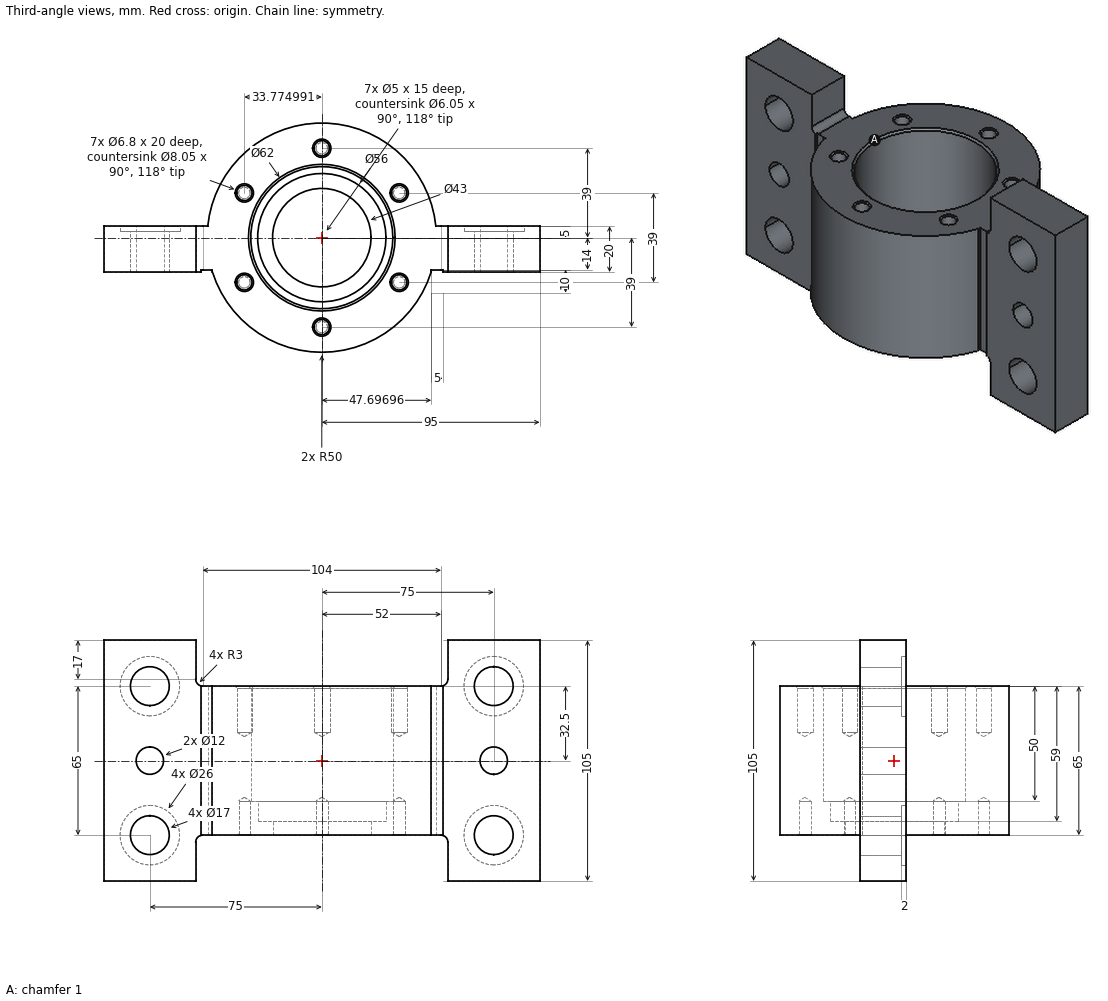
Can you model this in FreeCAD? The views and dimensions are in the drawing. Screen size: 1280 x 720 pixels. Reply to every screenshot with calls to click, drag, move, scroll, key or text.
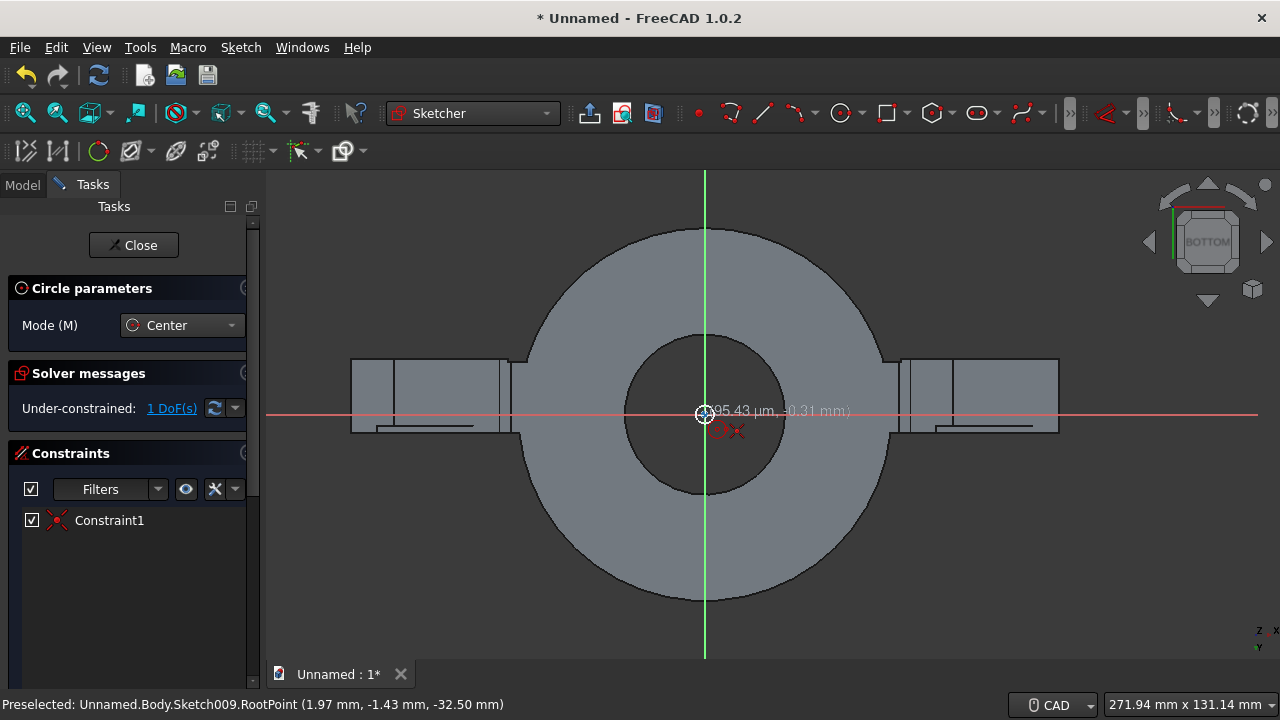
scroll(705, 560, up, 5)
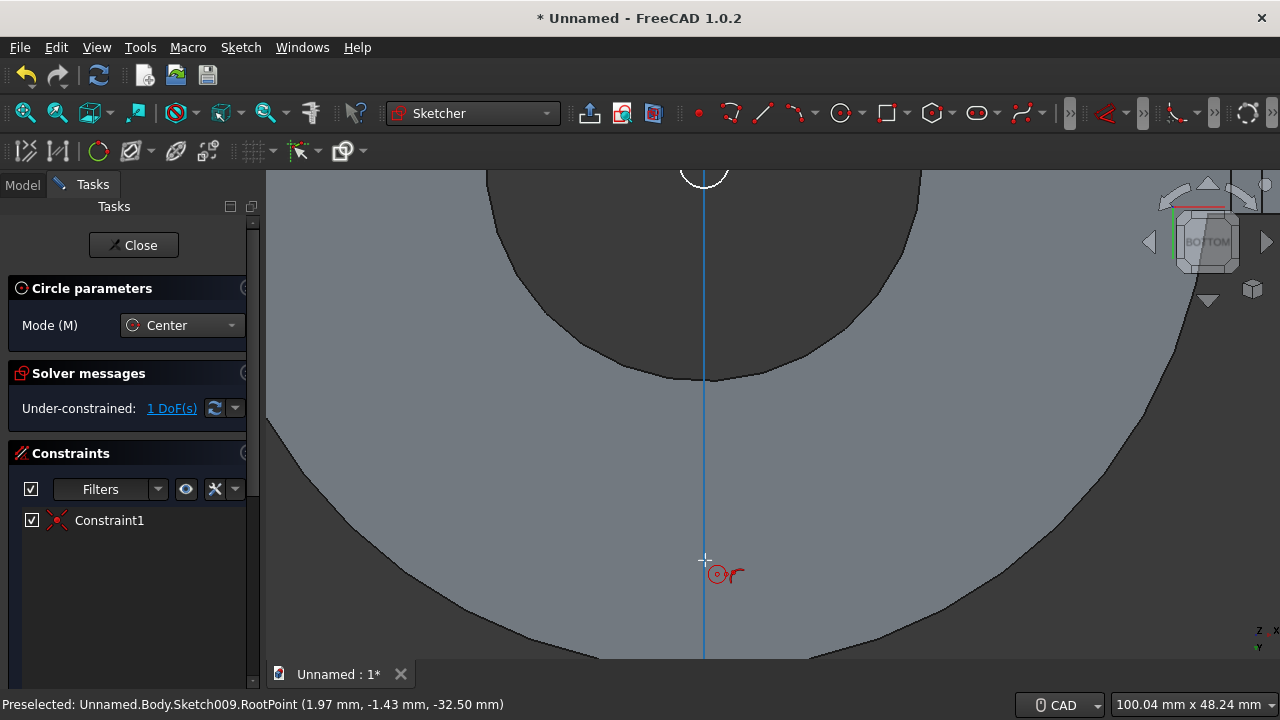
click(704, 559)
click(722, 541)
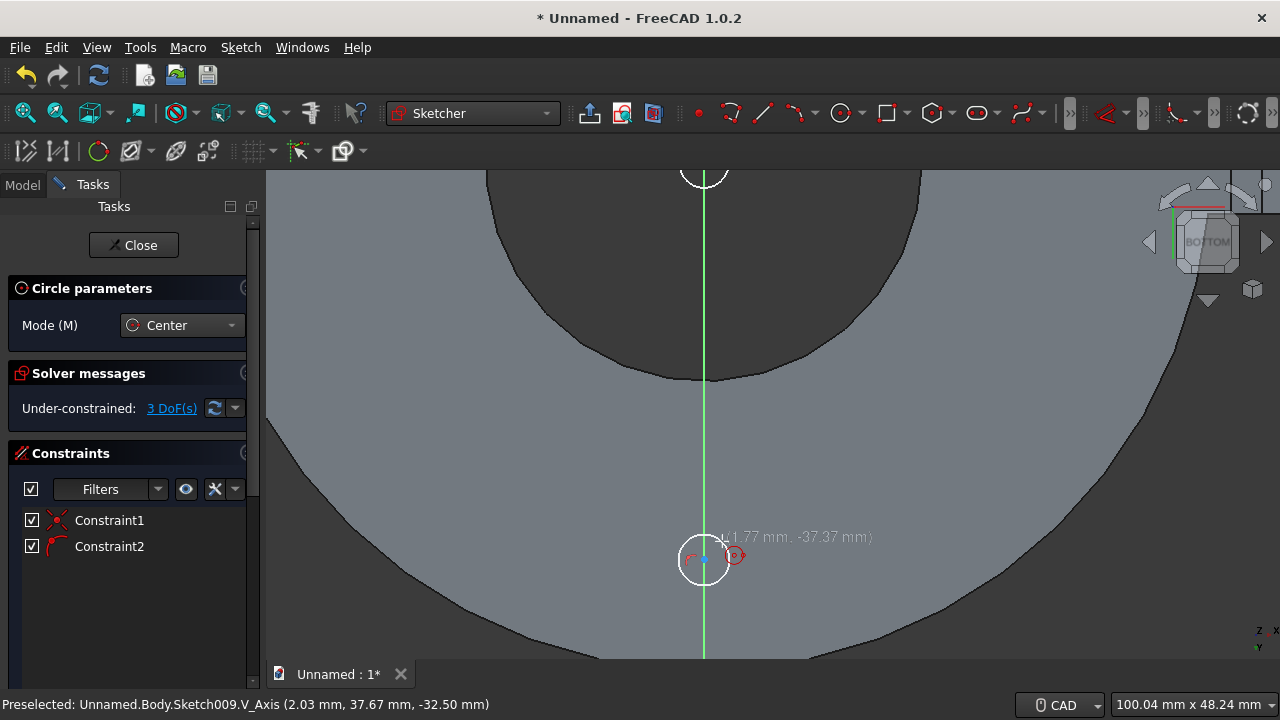
click(362, 361)
click(380, 343)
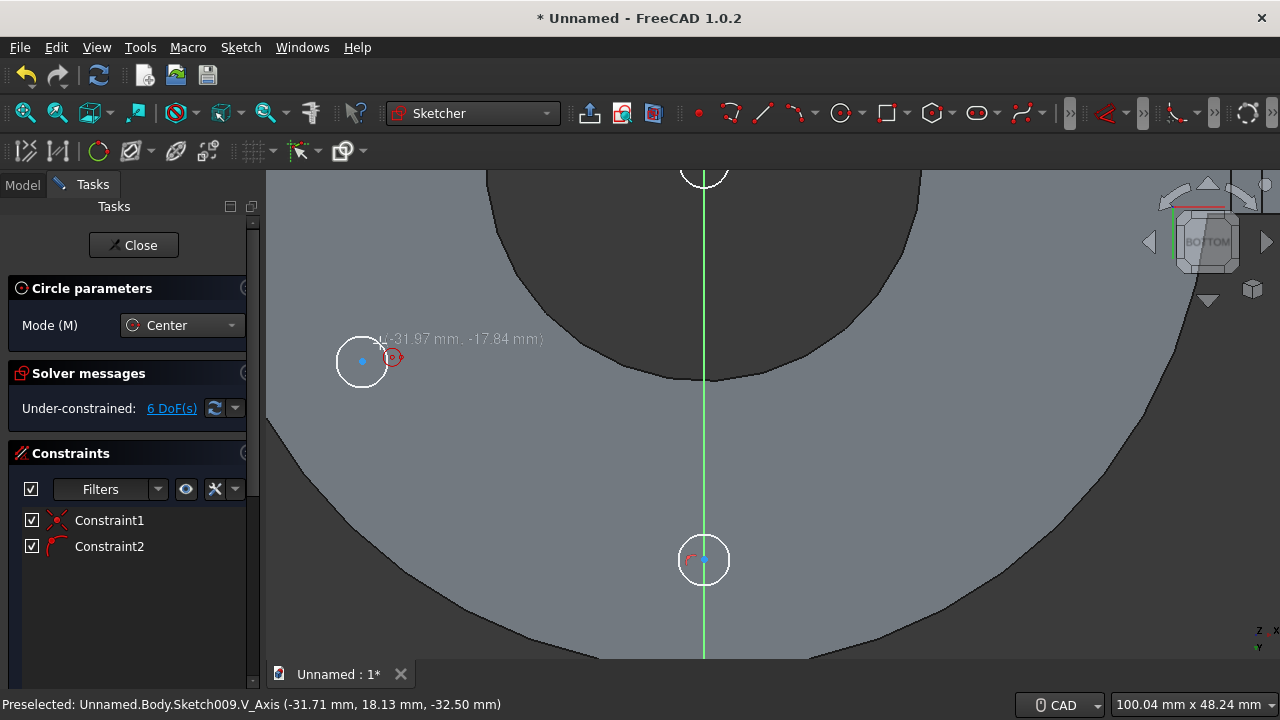
scroll(705, 561, down, 5)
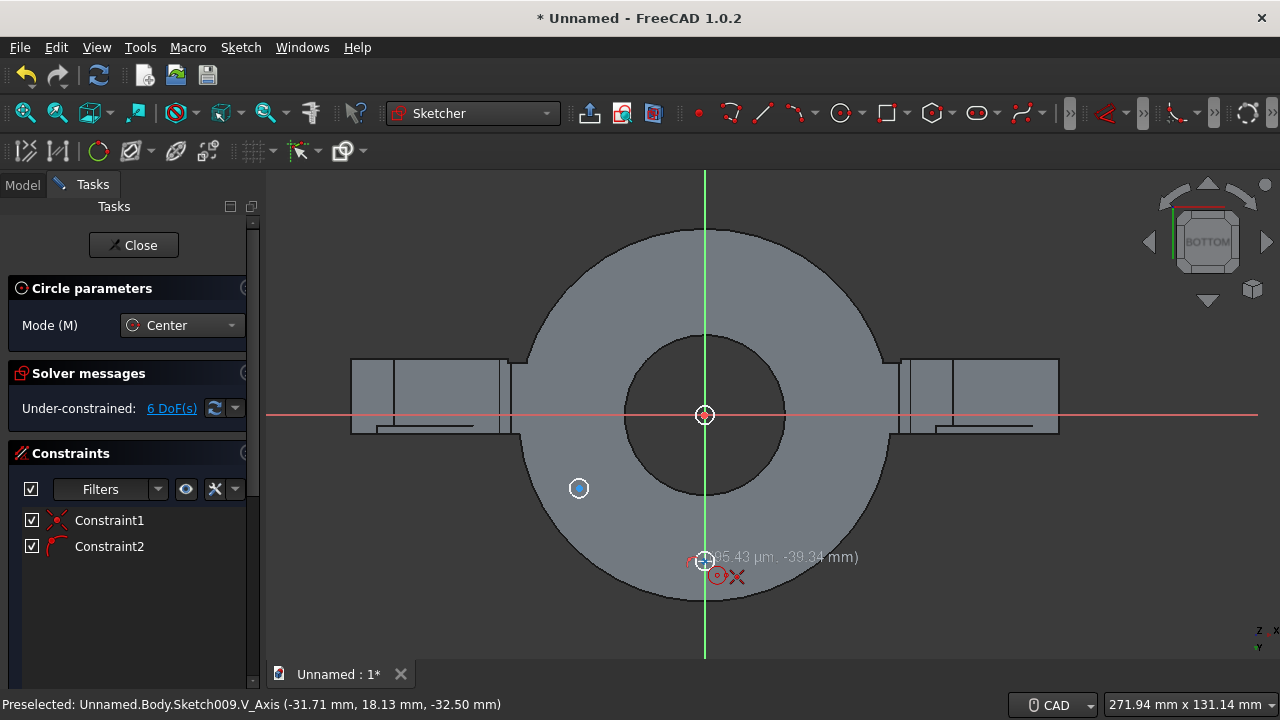
scroll(579, 342, up, 5)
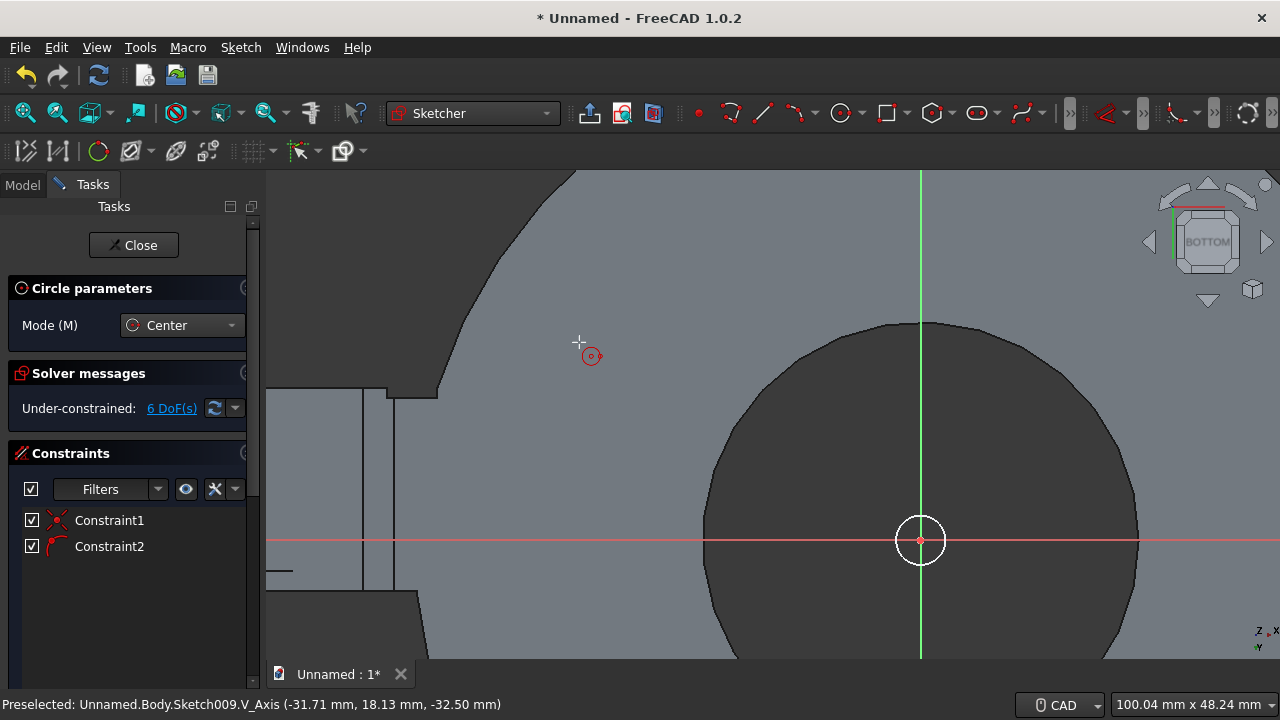
click(578, 343)
click(596, 325)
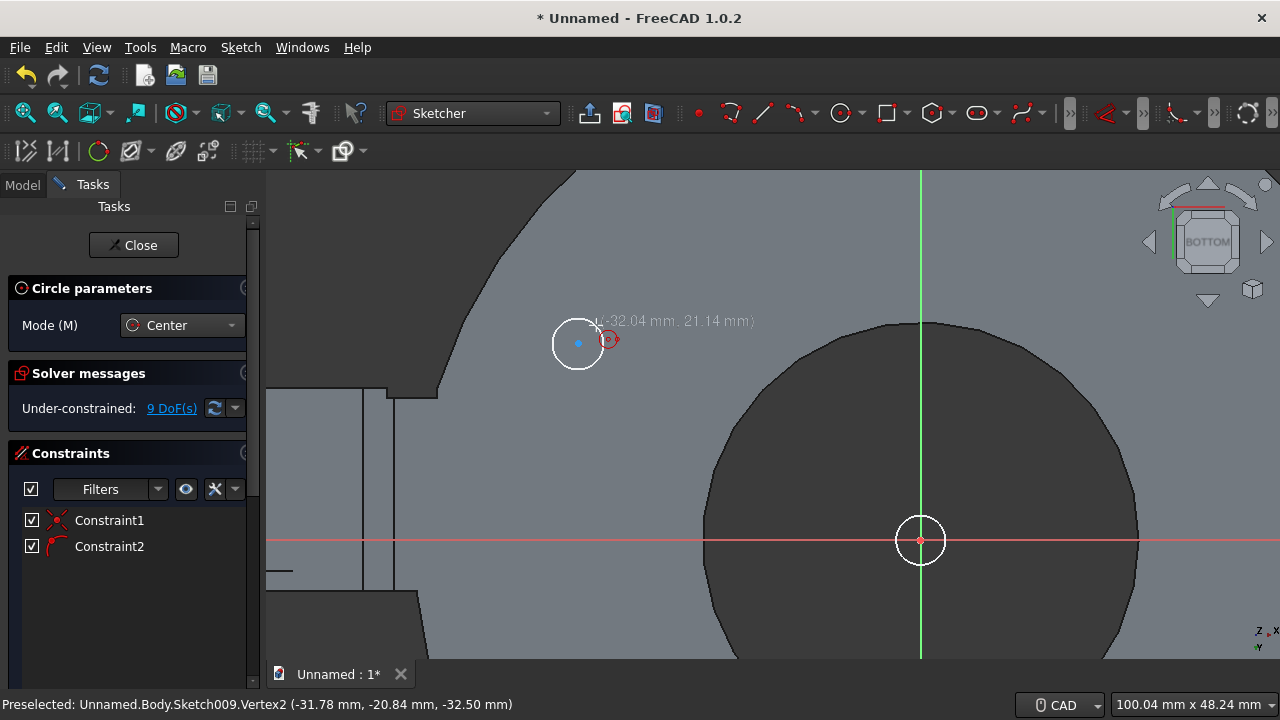
scroll(579, 341, down, 5)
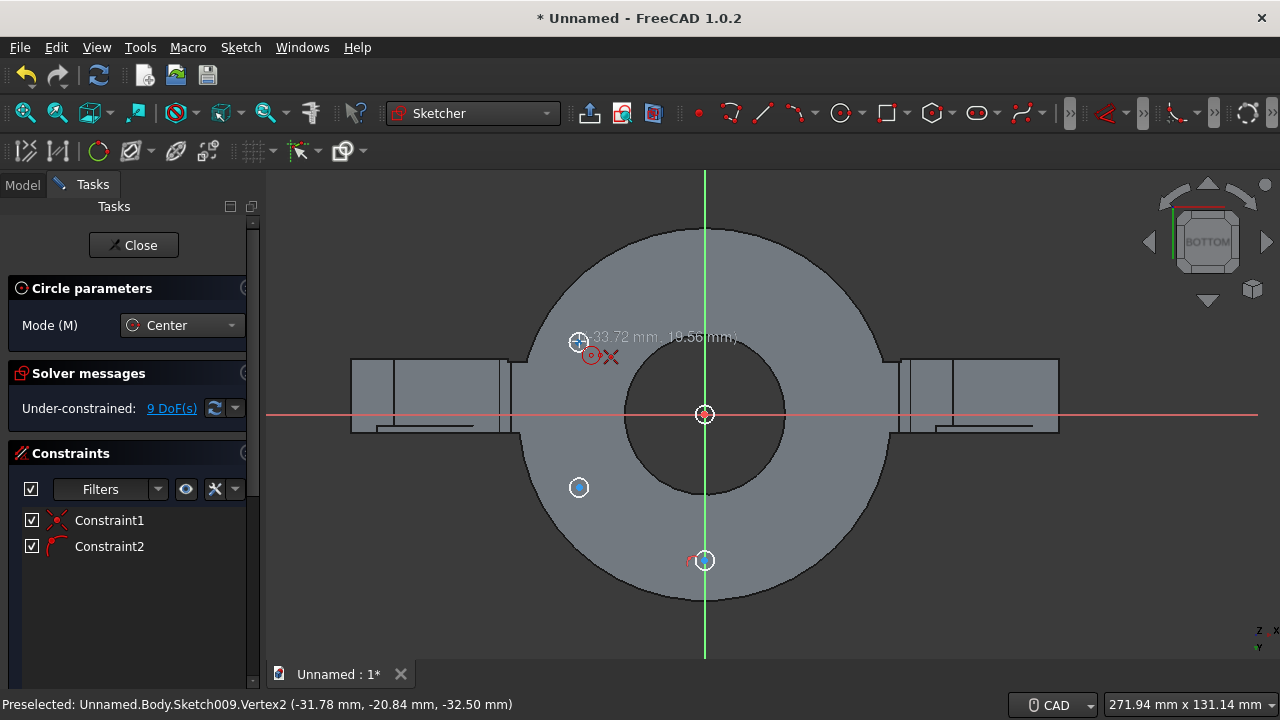
scroll(705, 269, up, 5)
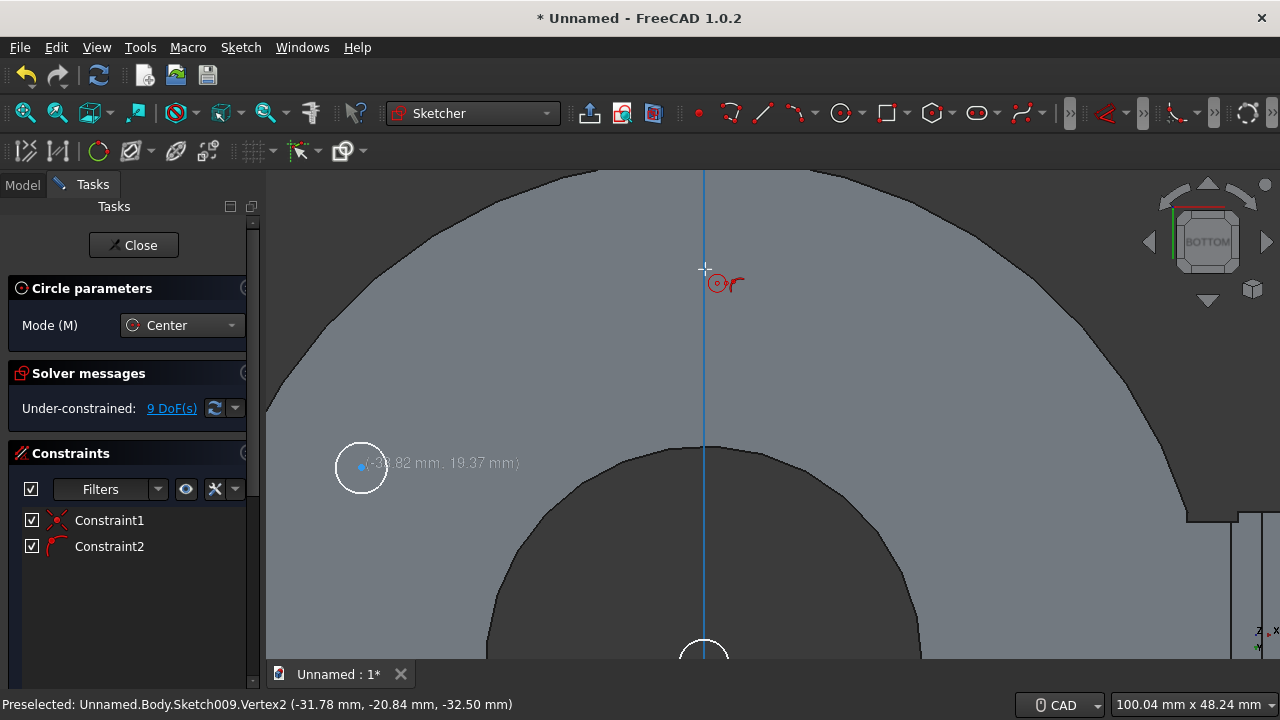
click(704, 269)
click(722, 251)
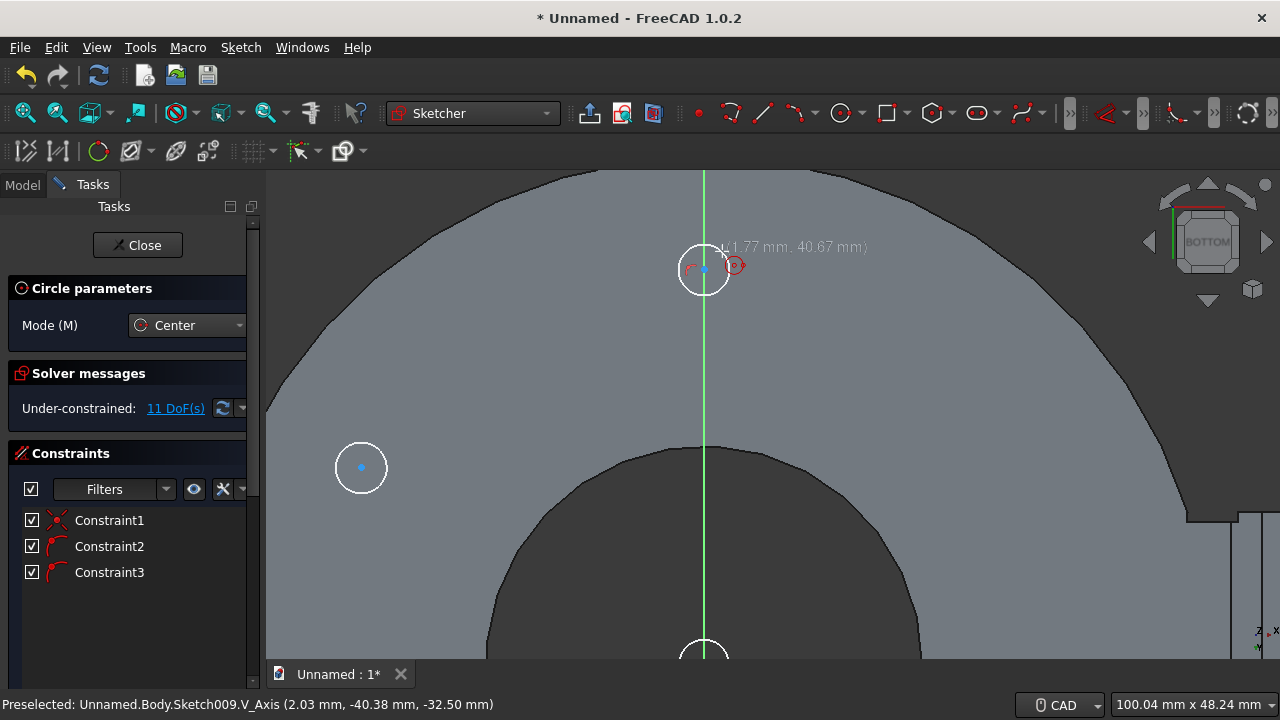
click(1046, 467)
click(1064, 449)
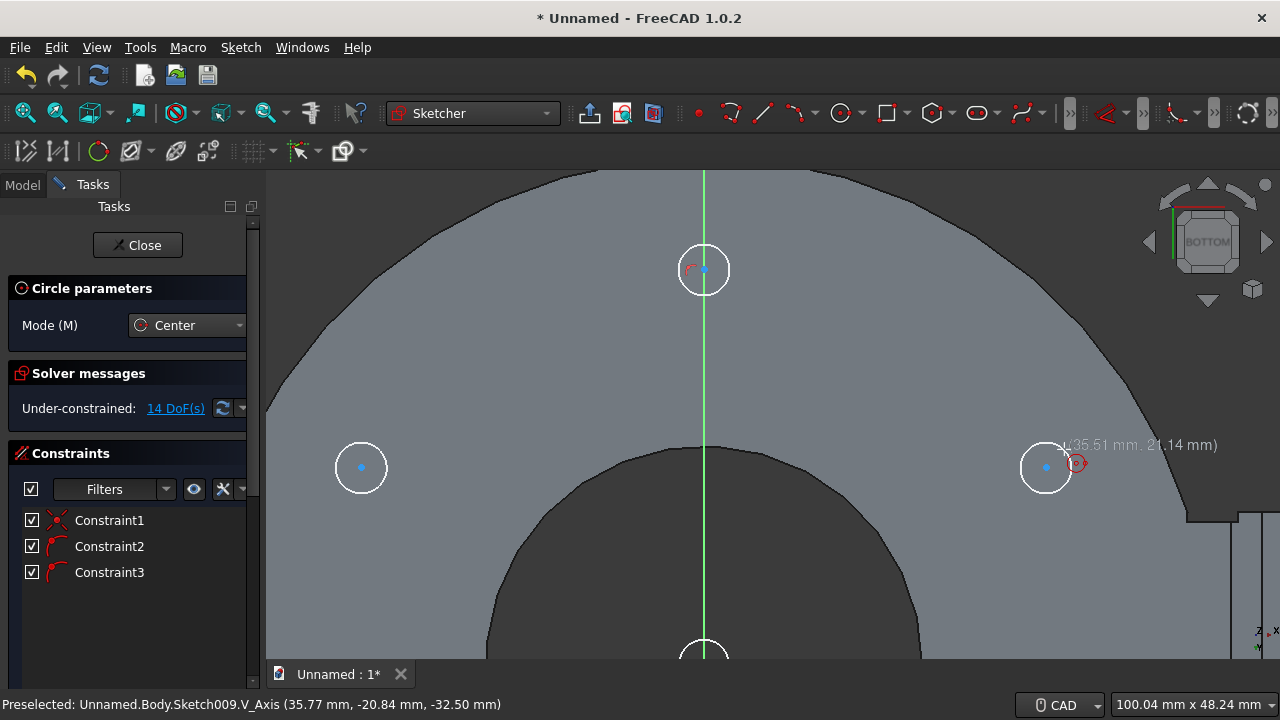
scroll(705, 269, down, 5)